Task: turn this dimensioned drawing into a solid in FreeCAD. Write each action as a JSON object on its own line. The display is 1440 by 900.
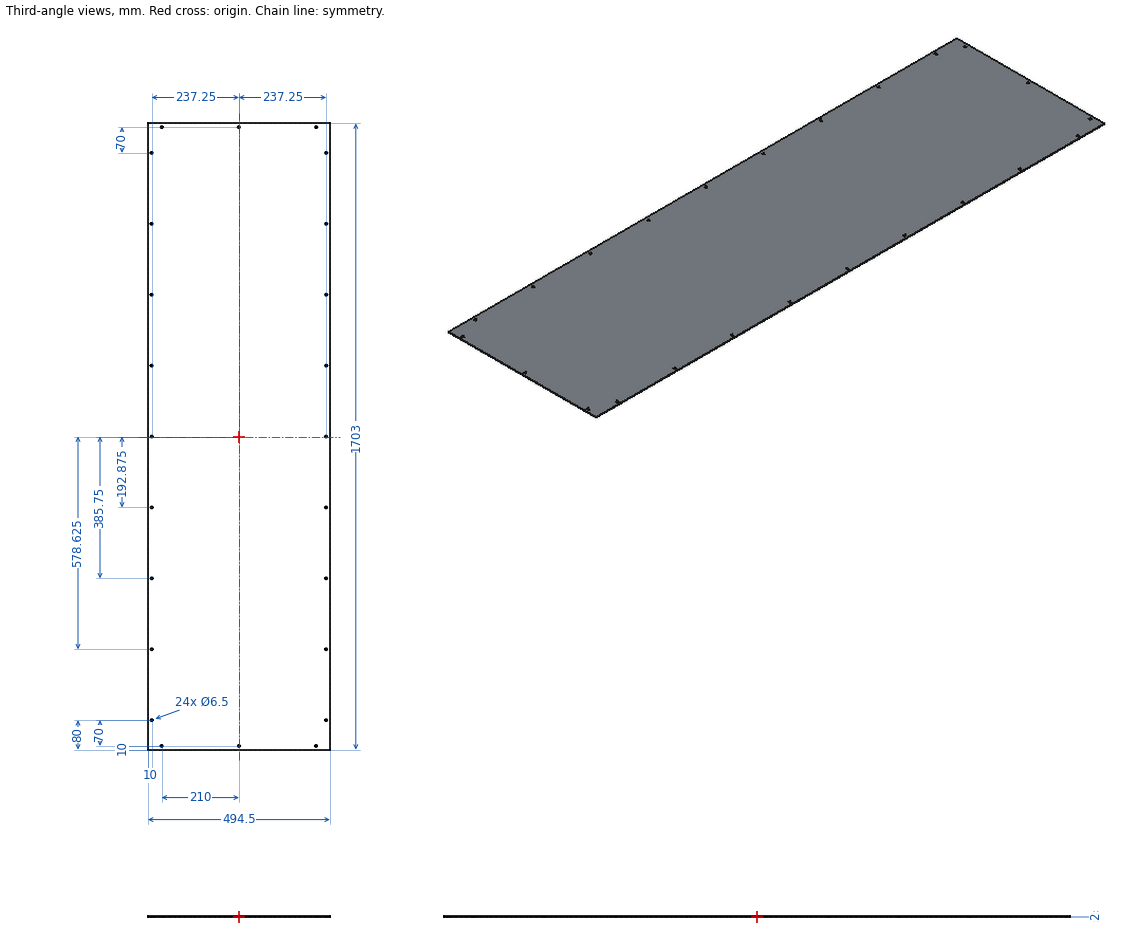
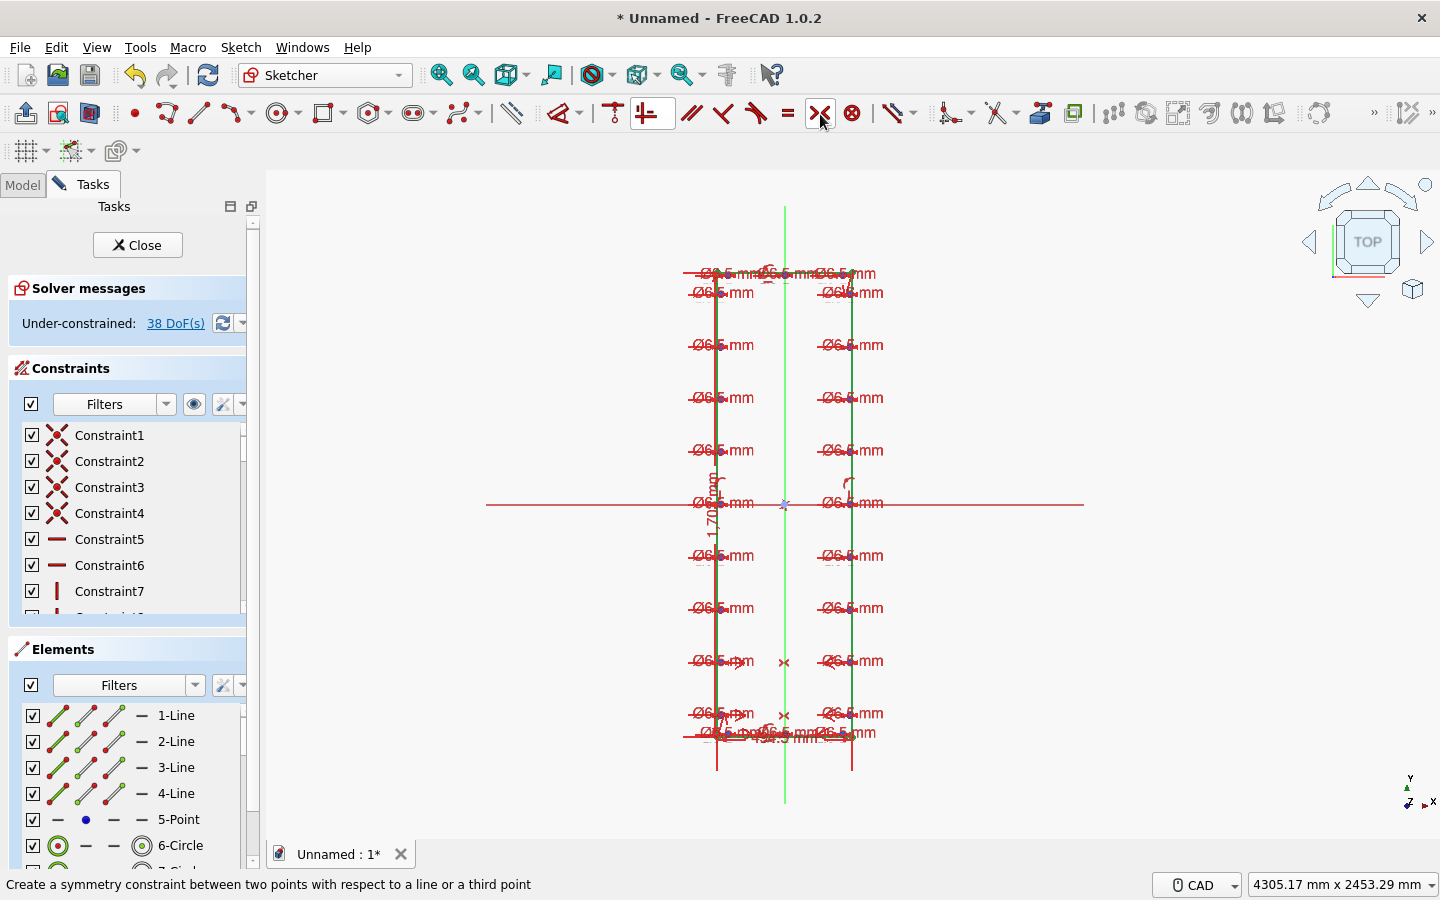
{"action": "left_click", "coordinate": [720, 610]}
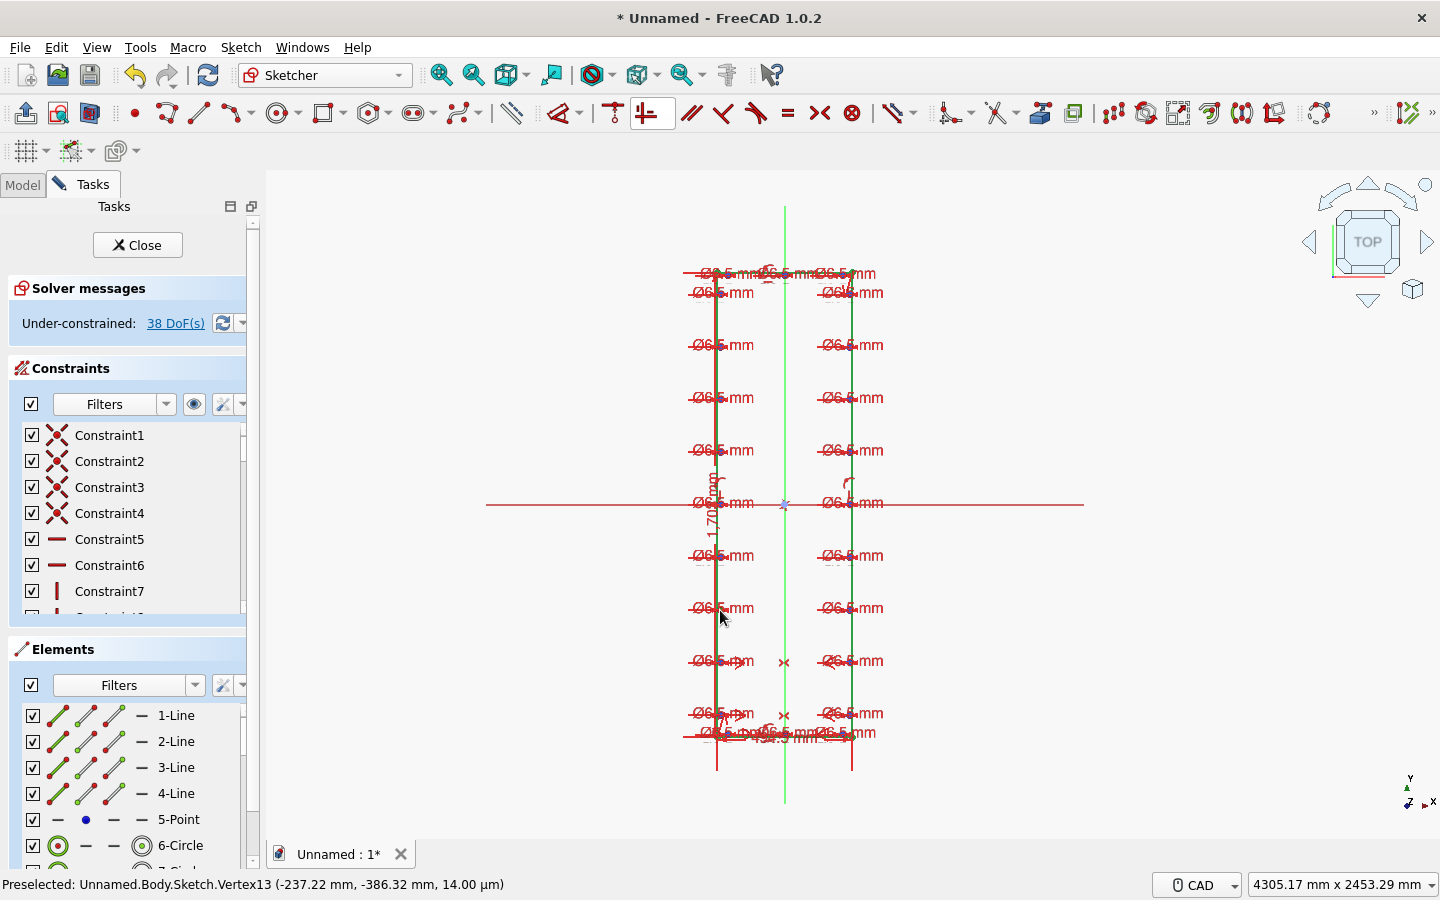
{"action": "left_click", "coordinate": [850, 610]}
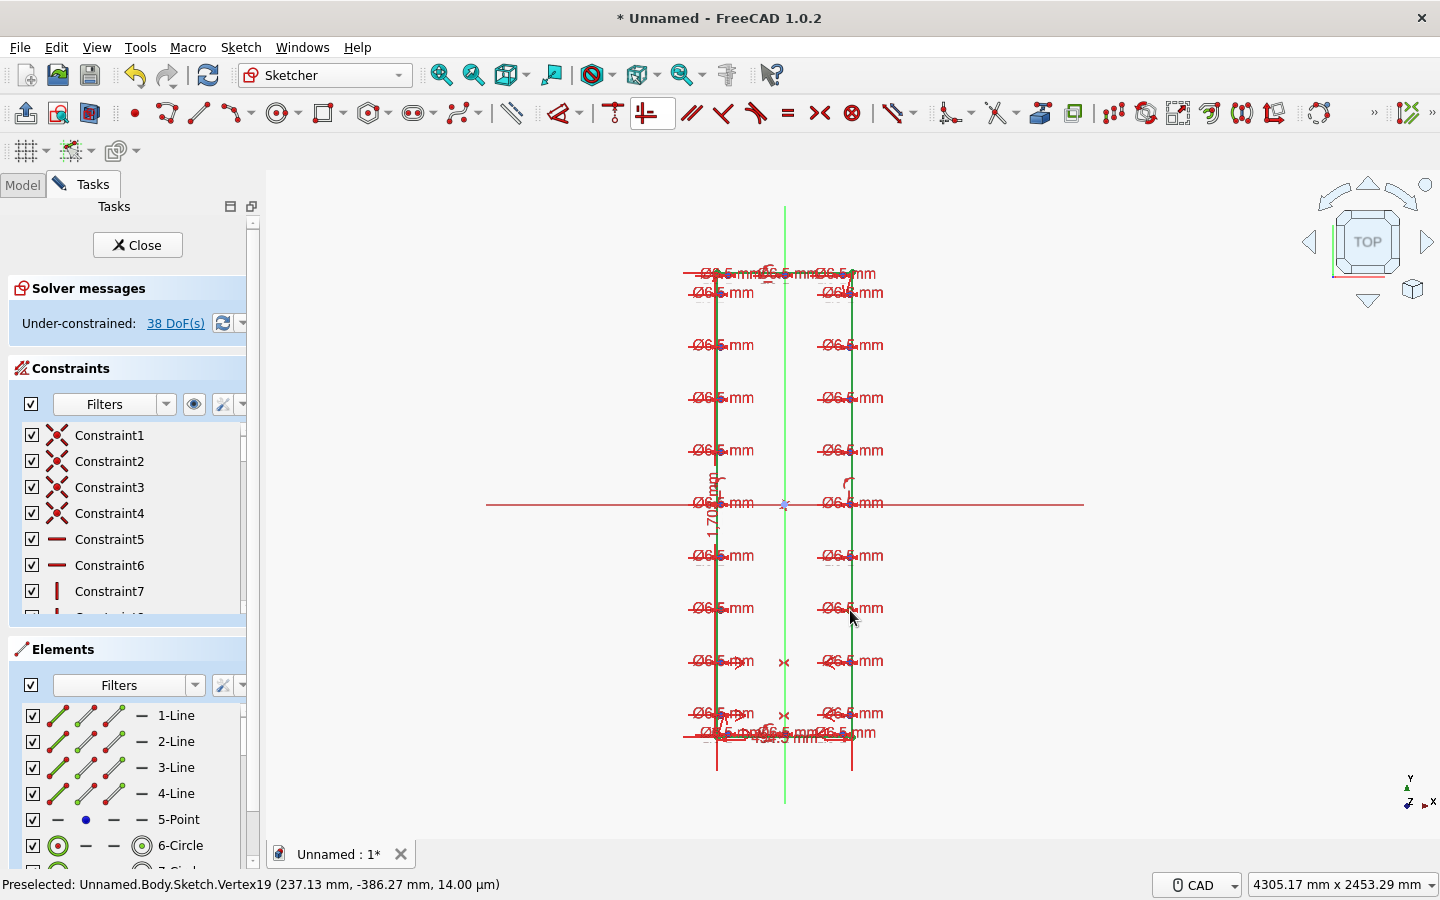
{"action": "left_click", "coordinate": [785, 767]}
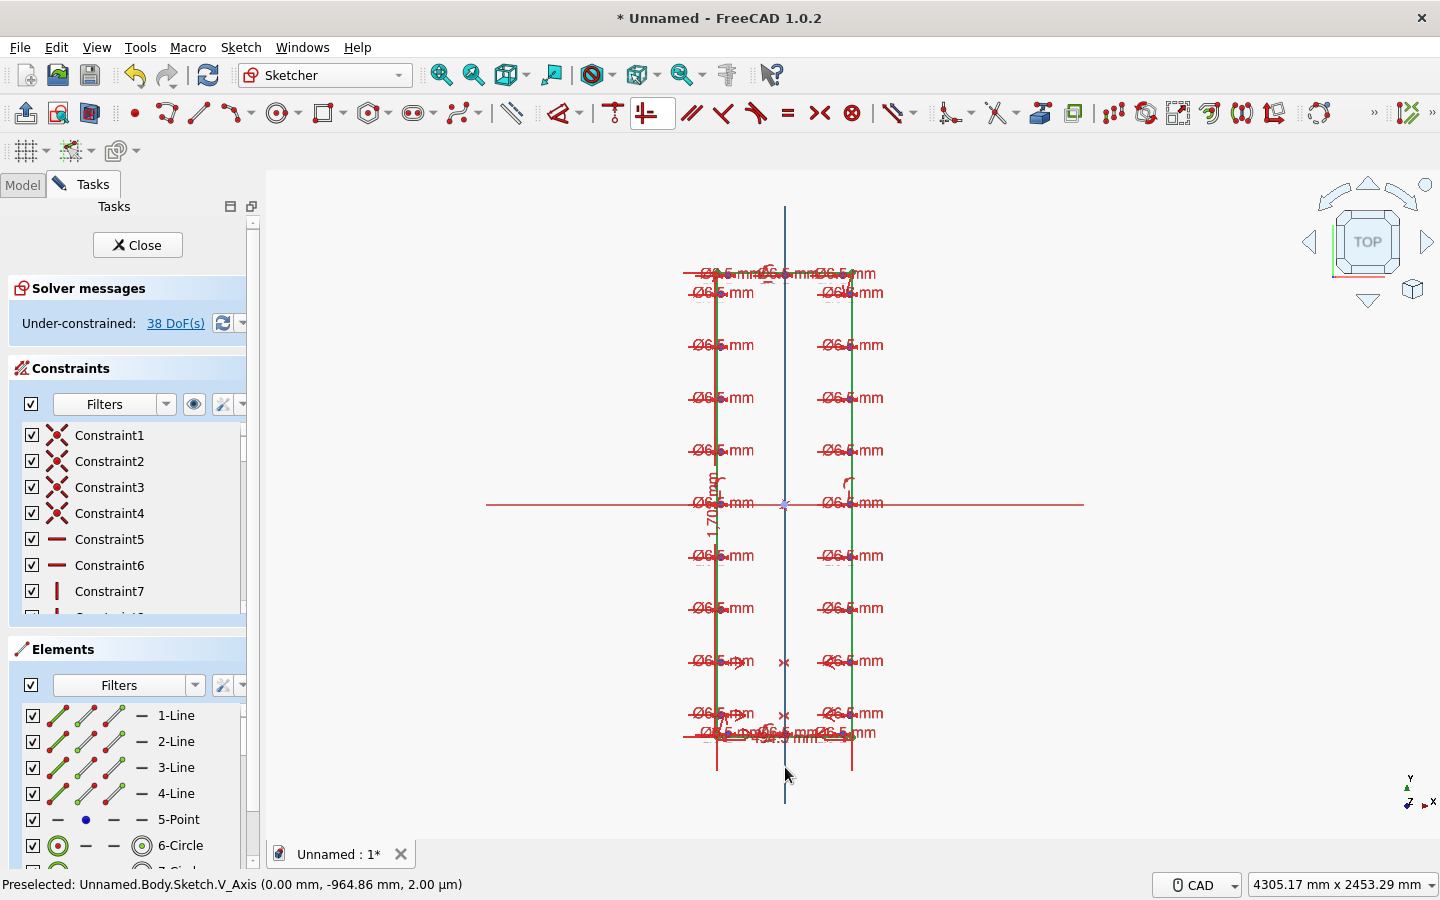
{"action": "left_click", "coordinate": [820, 114]}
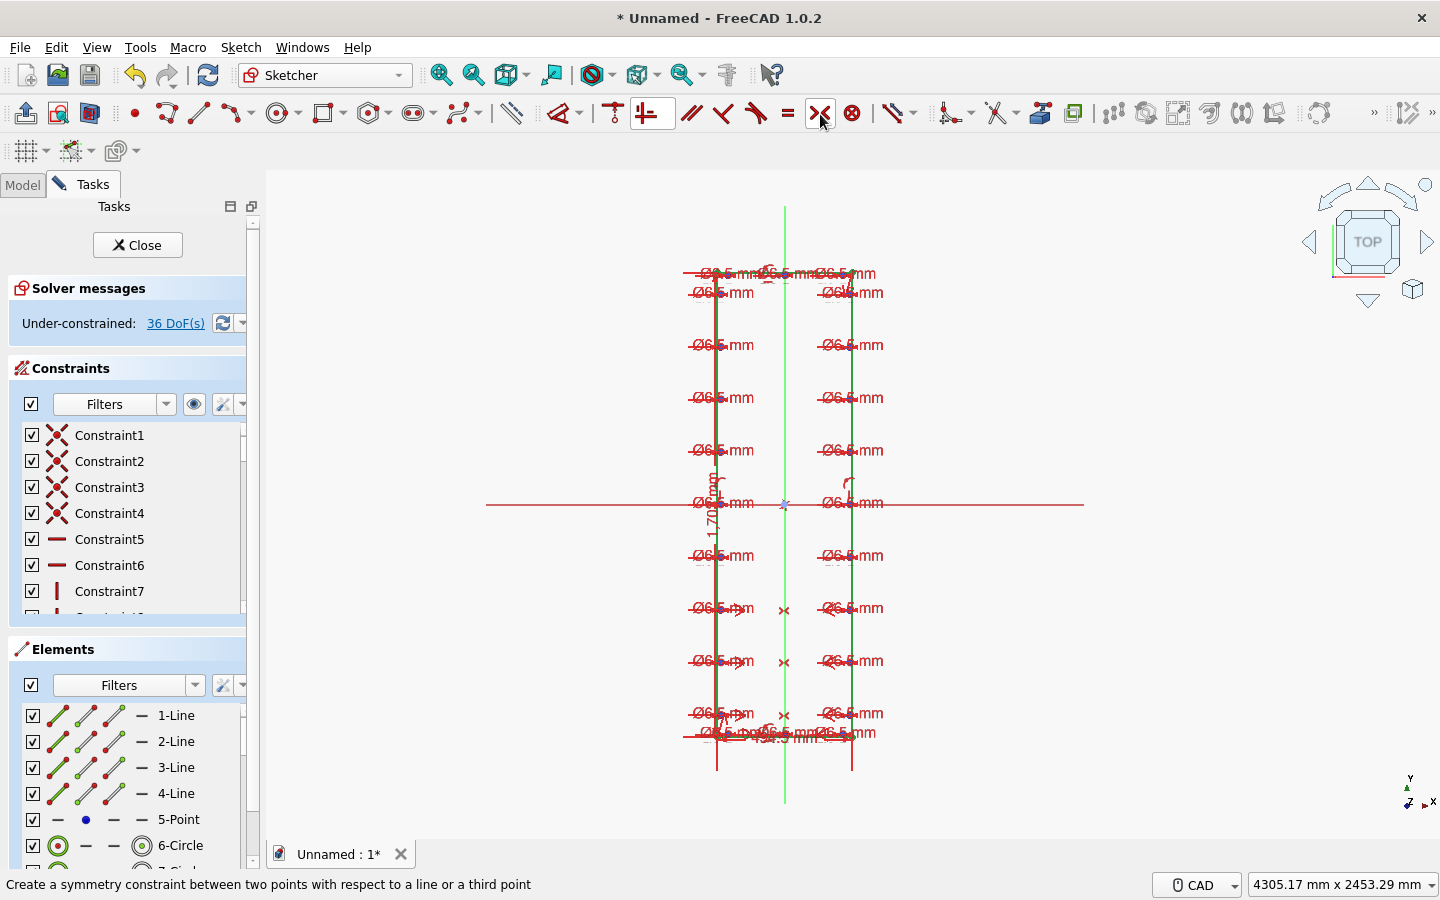
{"action": "left_click", "coordinate": [720, 558]}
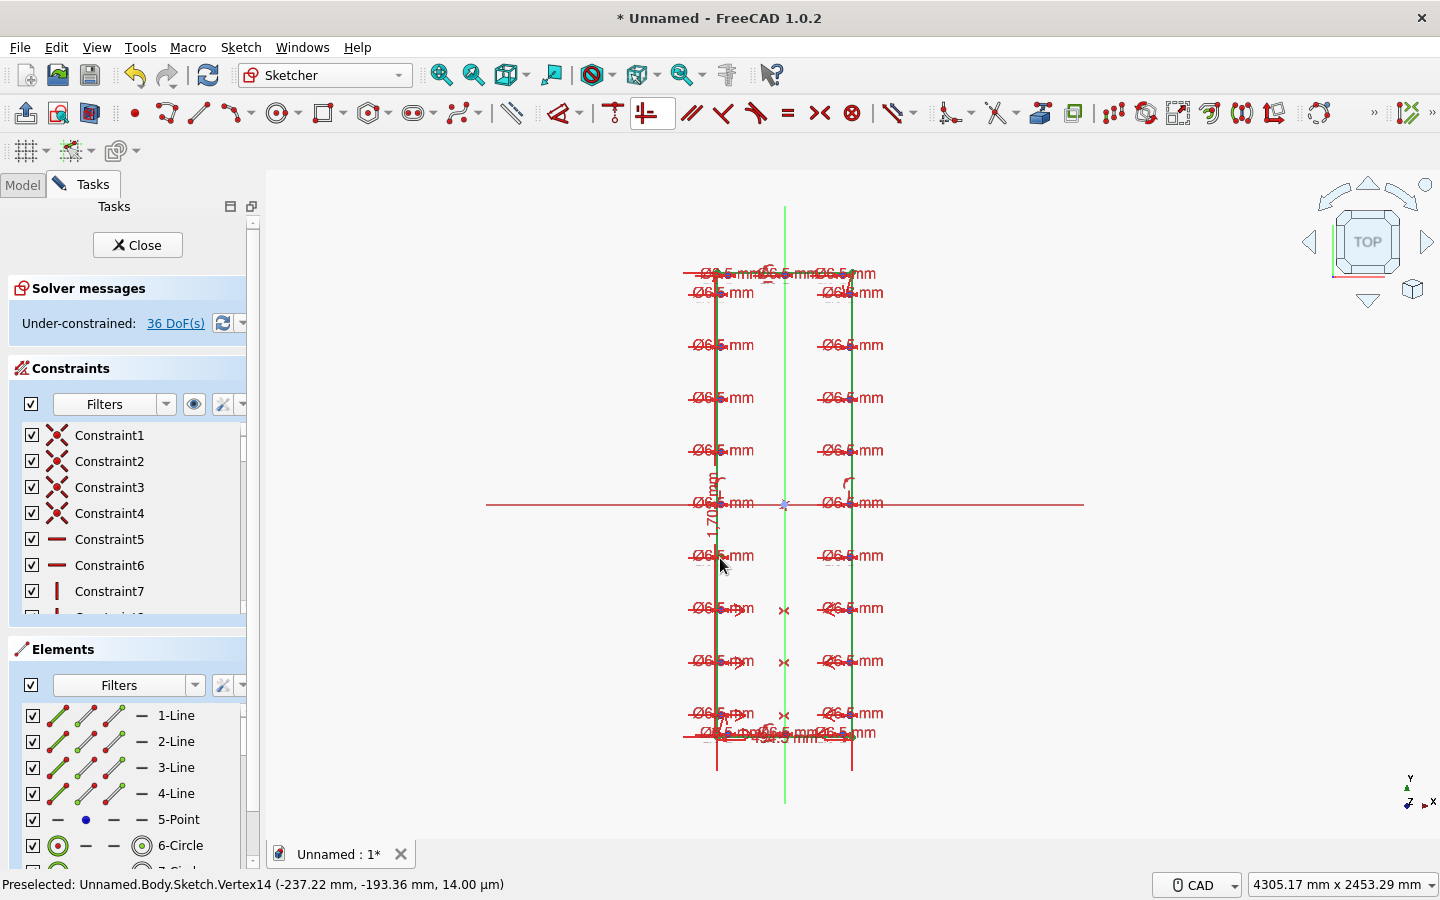
{"action": "left_click", "coordinate": [850, 558]}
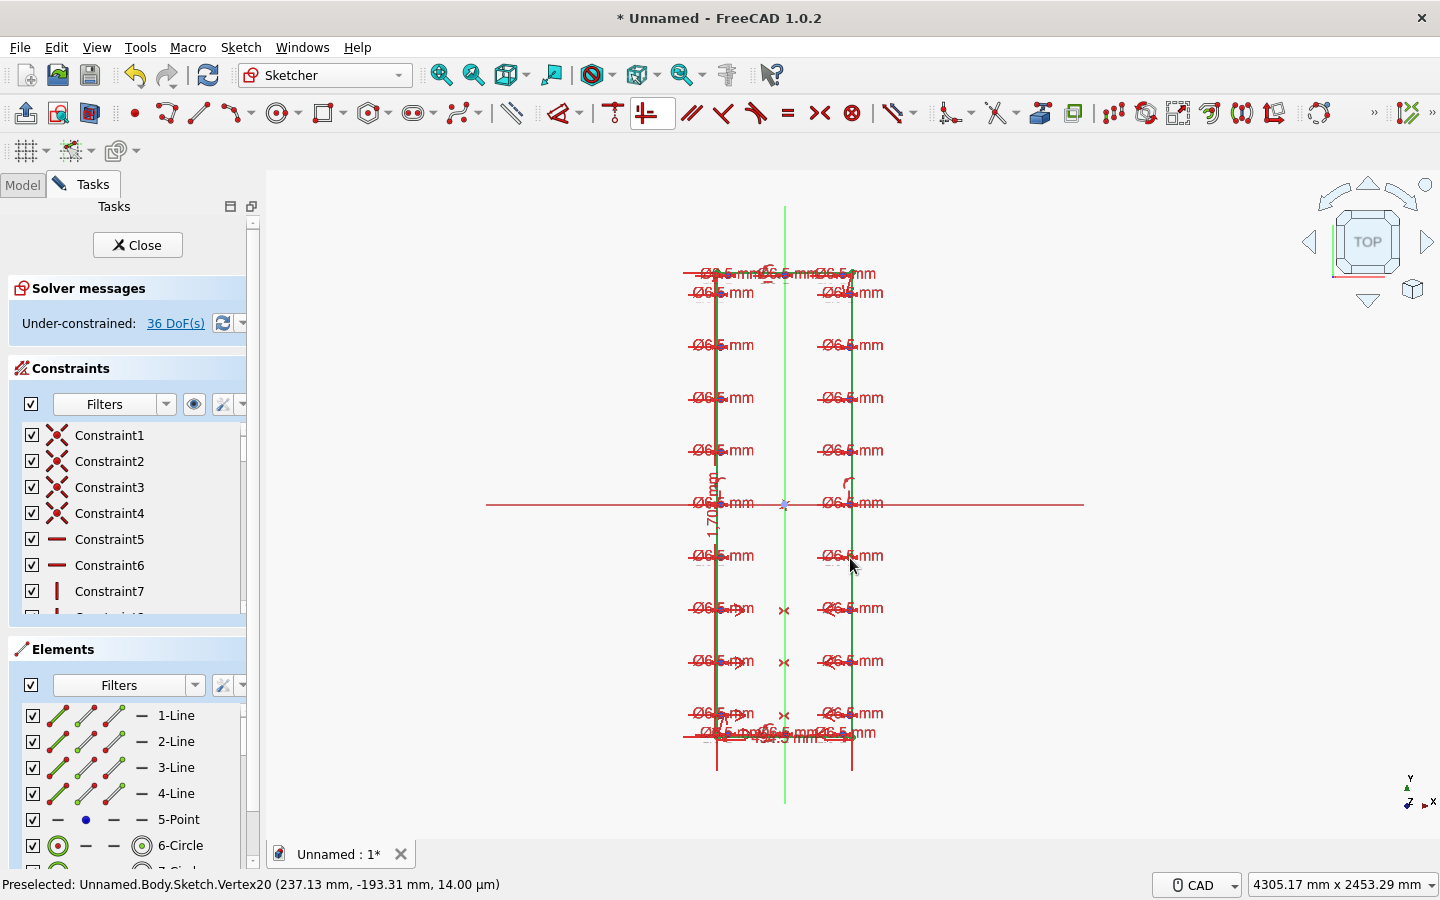
{"action": "left_click", "coordinate": [785, 767]}